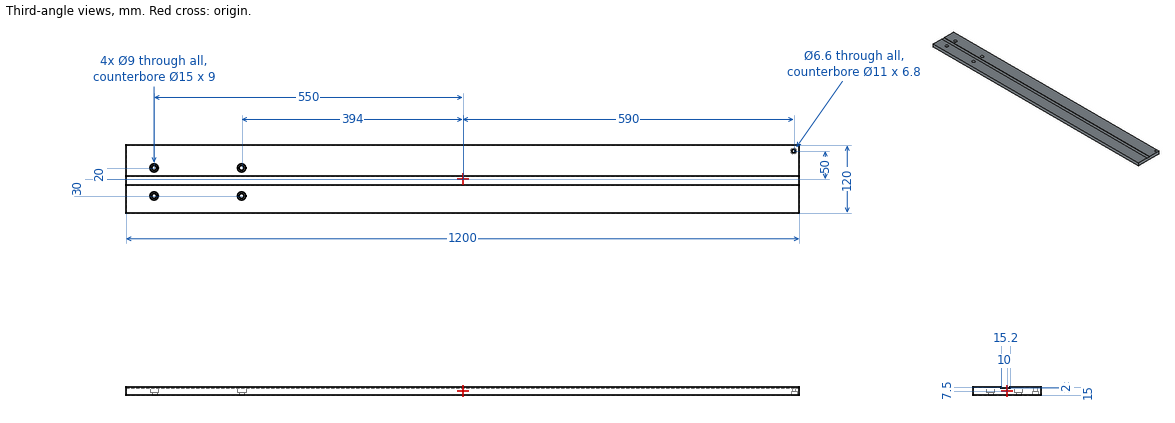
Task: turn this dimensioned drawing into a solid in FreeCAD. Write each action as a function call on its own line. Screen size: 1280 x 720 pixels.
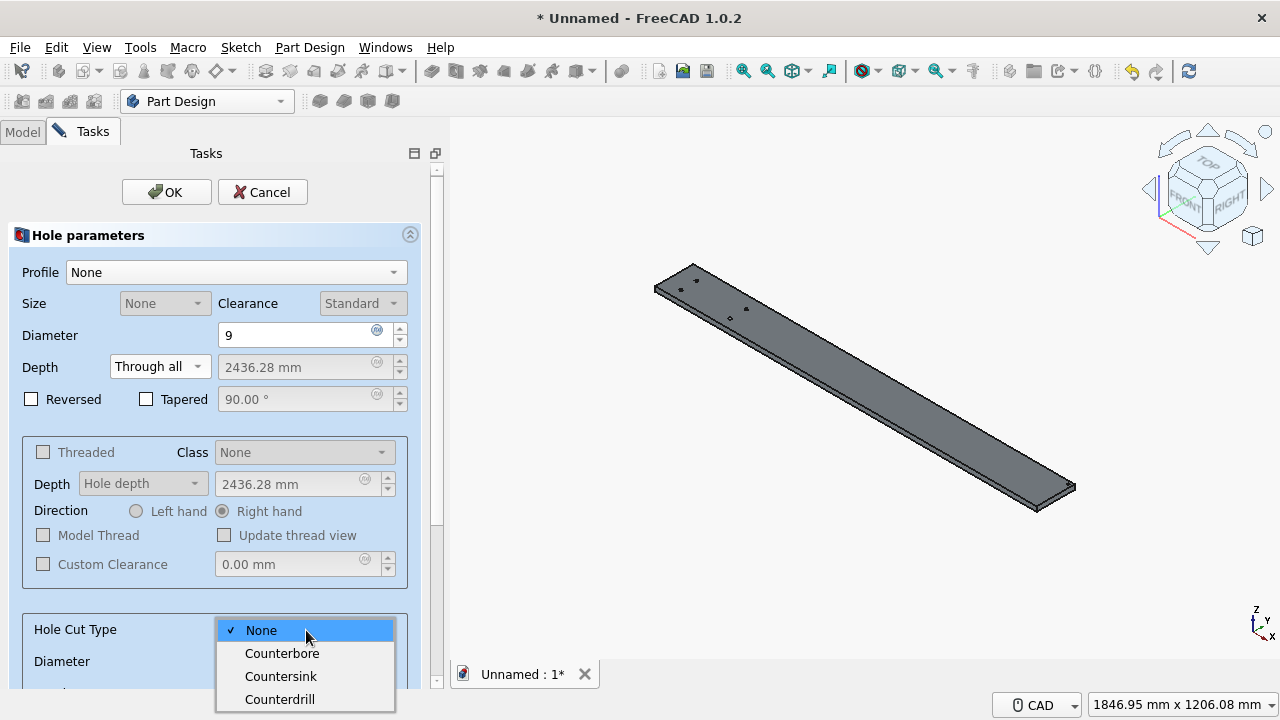
click(304, 654)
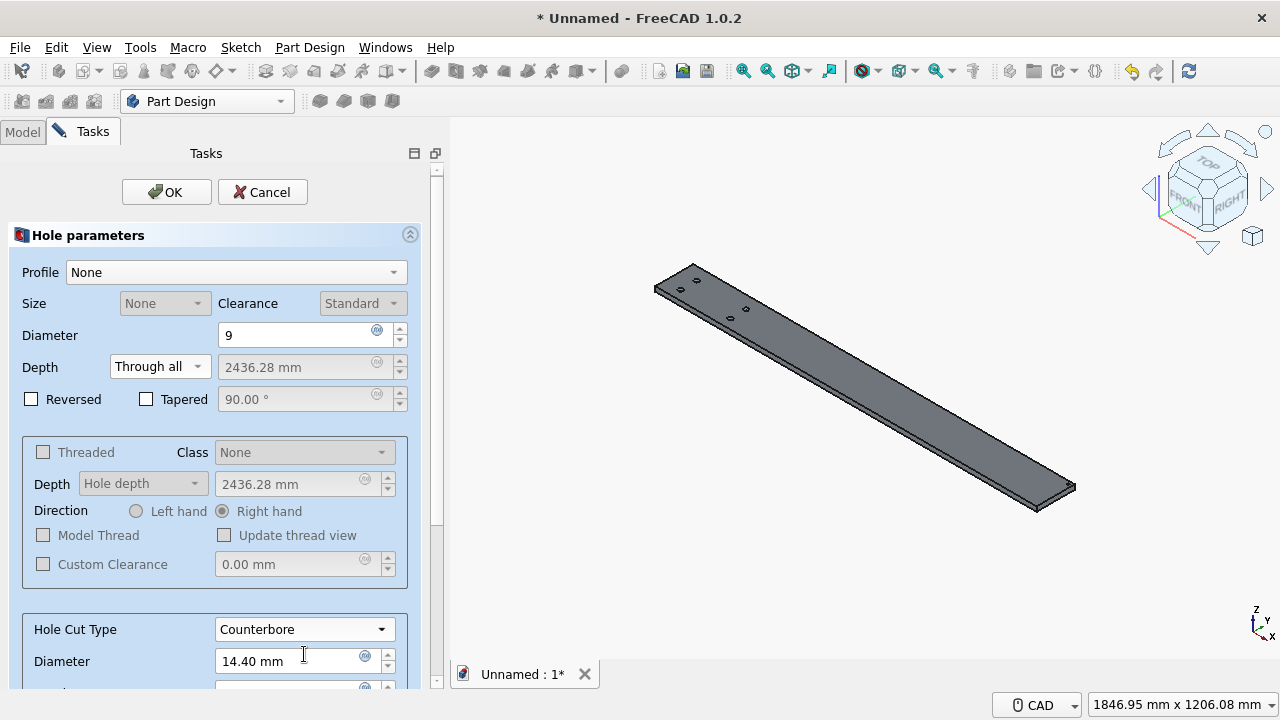
triple_click(298, 661)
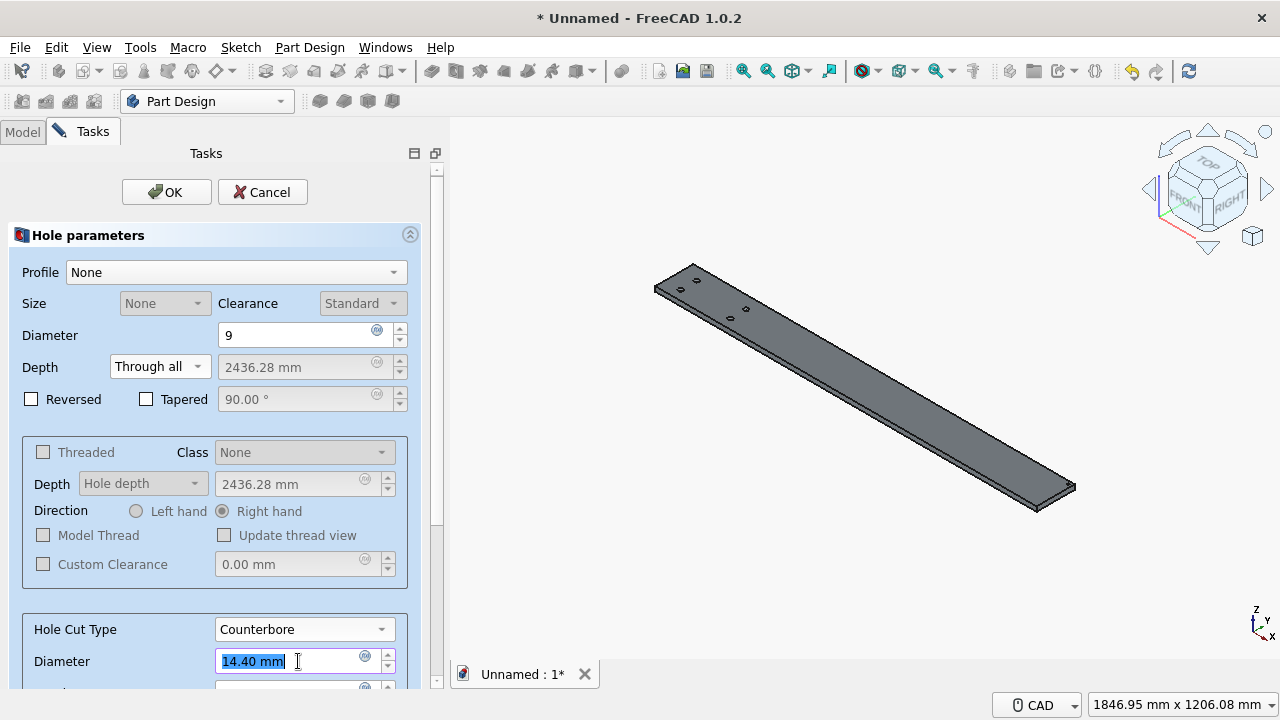
text(15)
key(Tab)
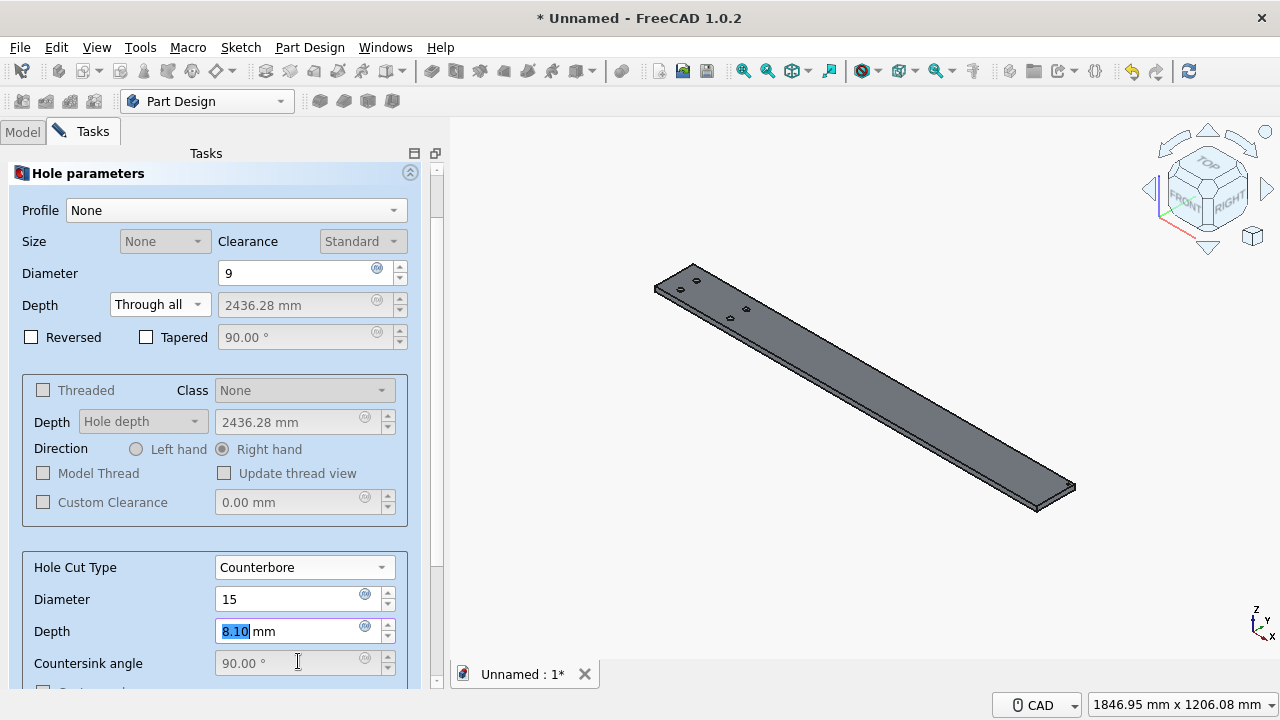
text(9)
key(Tab)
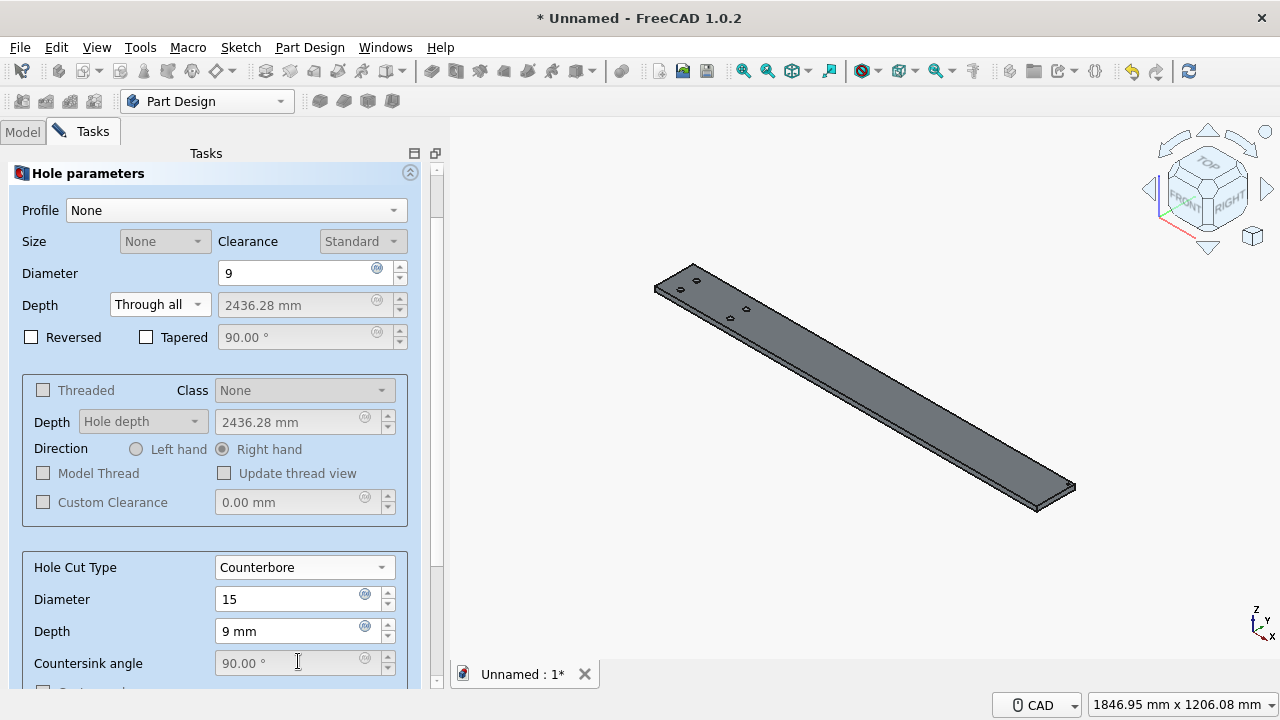
scroll(437, 426, up, 2)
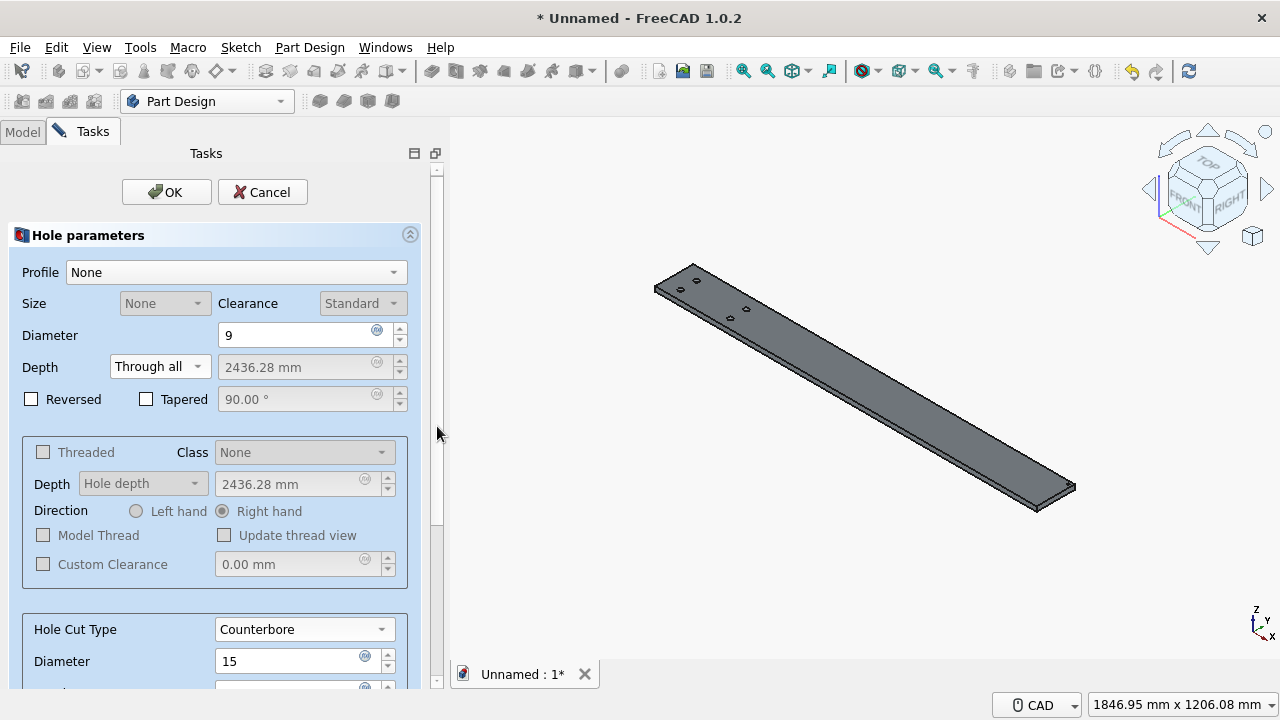
click(167, 192)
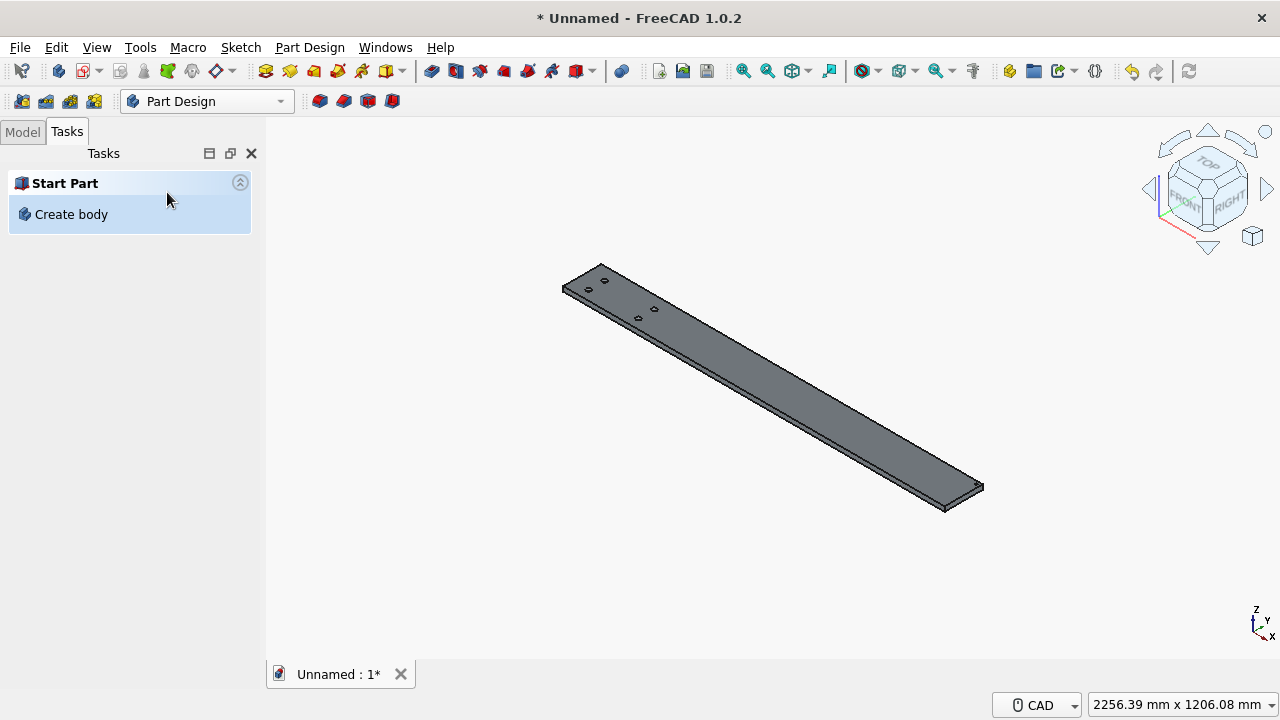
scroll(980, 488, up, 7)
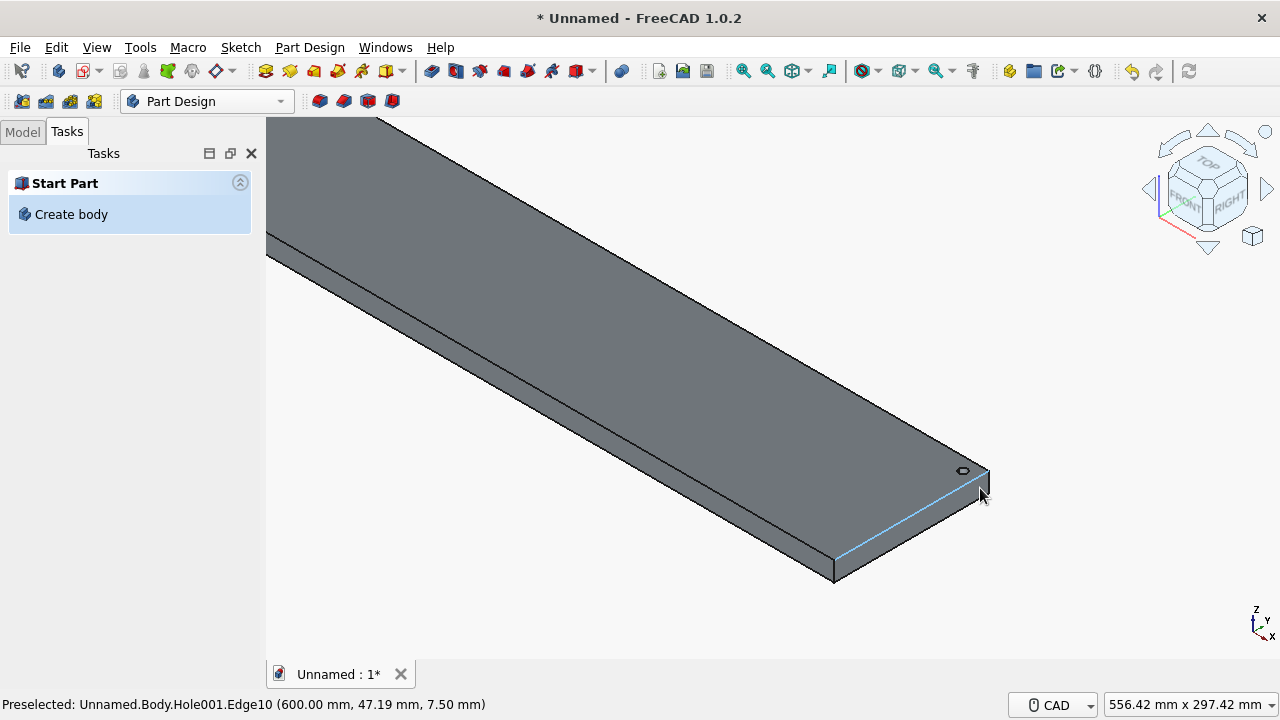
click(978, 488)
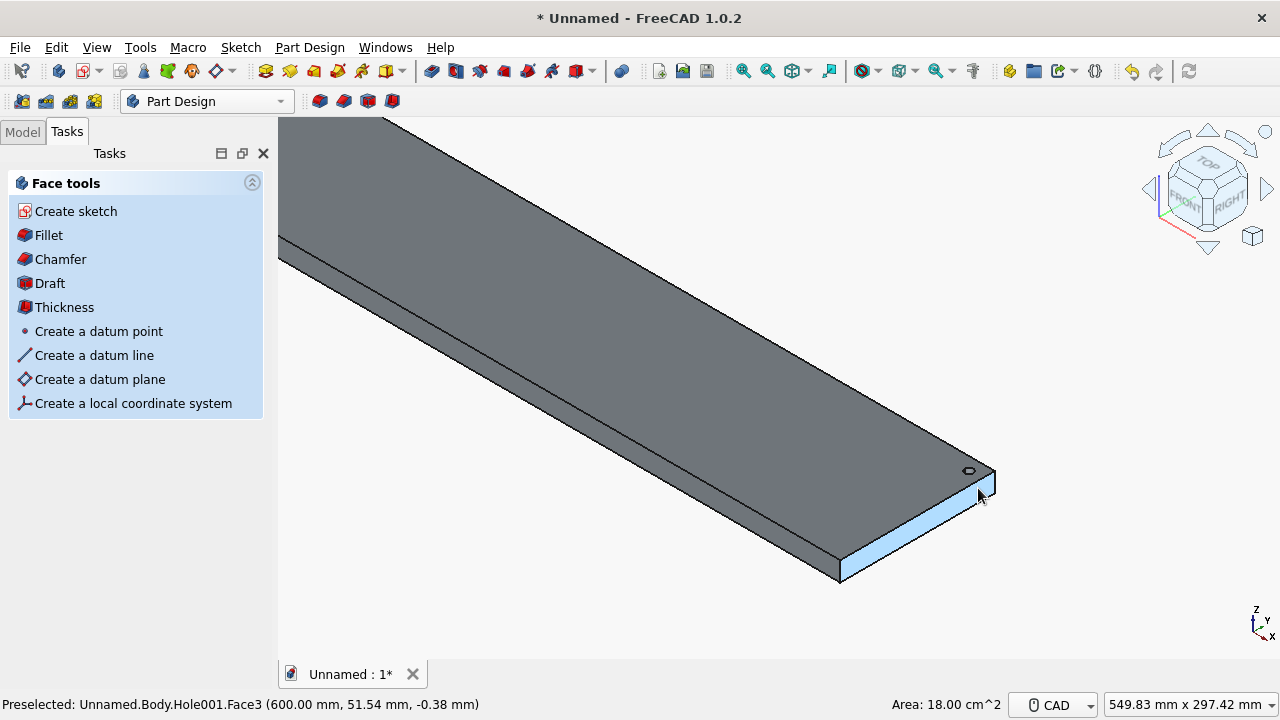
click(84, 72)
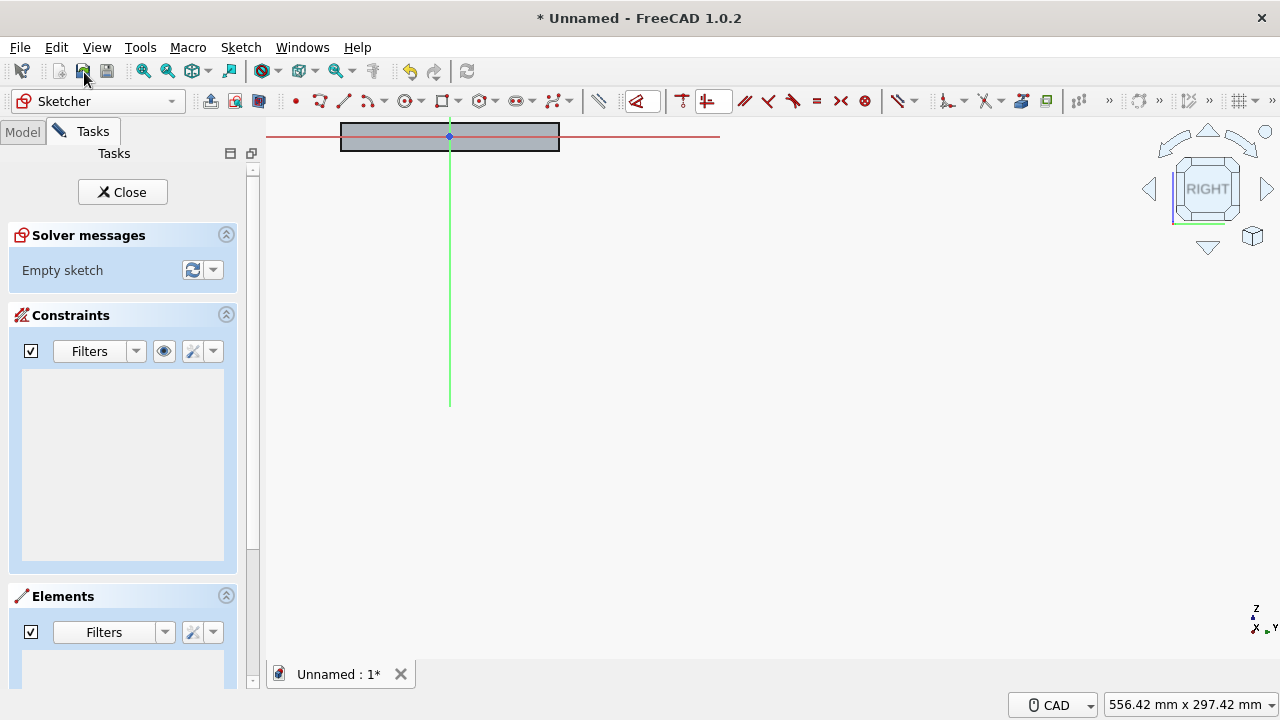
scroll(704, 388, down, 5)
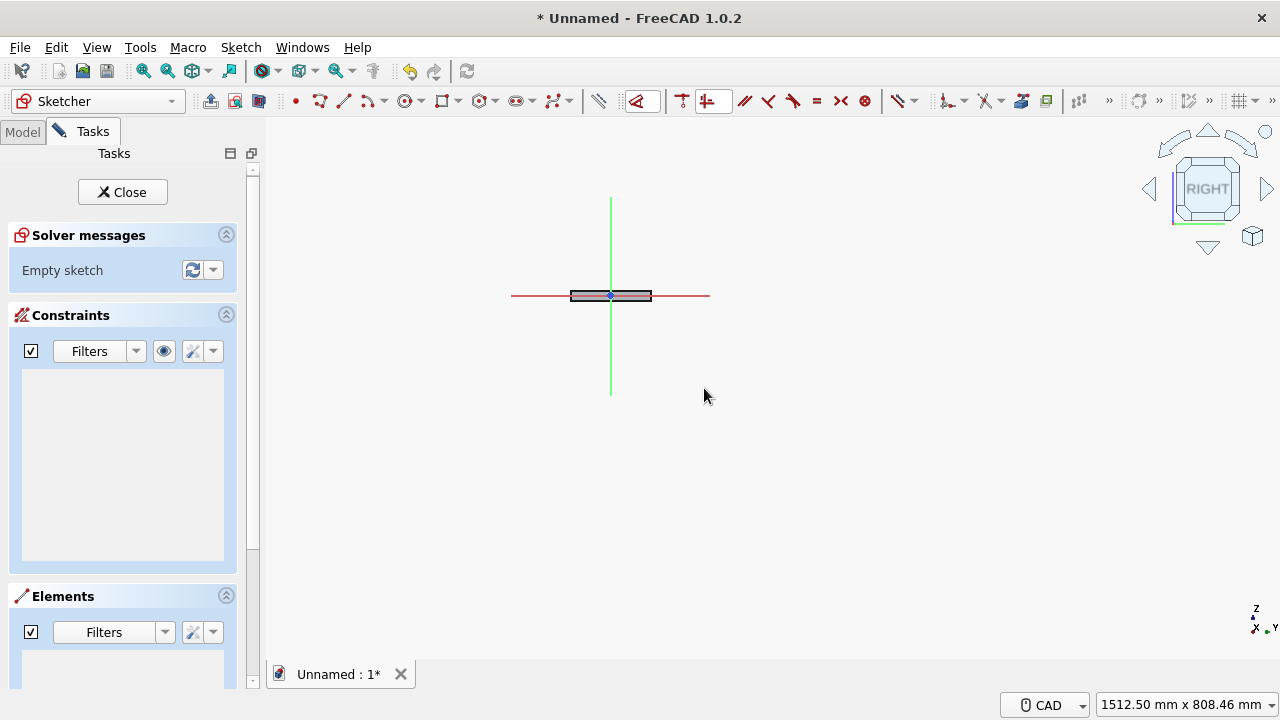
scroll(604, 288, up, 15)